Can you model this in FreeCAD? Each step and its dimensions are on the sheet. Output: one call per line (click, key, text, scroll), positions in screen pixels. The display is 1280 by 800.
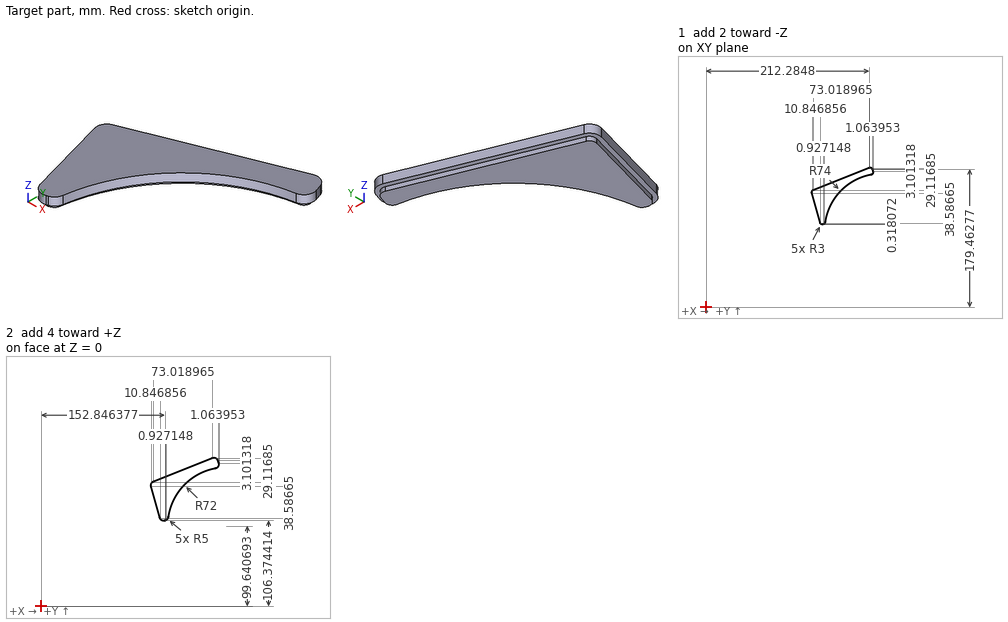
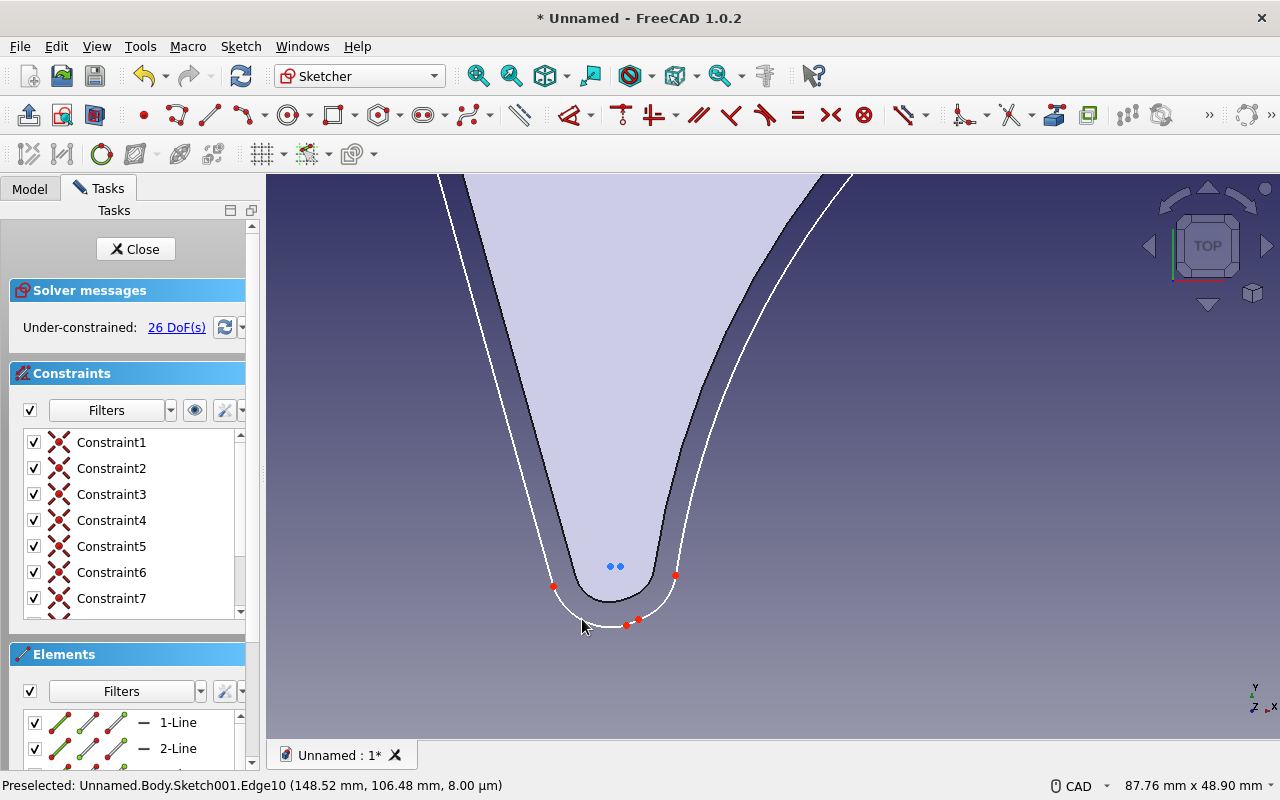
scroll(633, 622, up, 4)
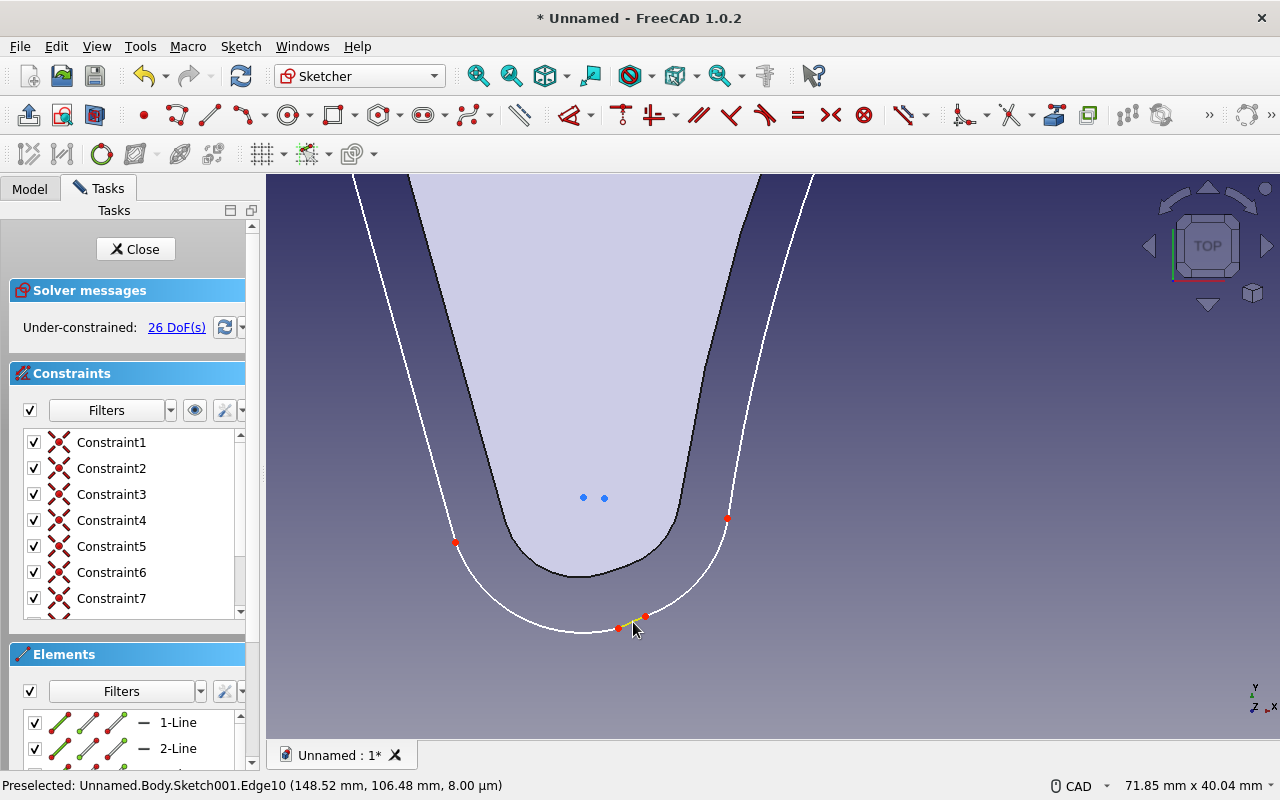
click(632, 622)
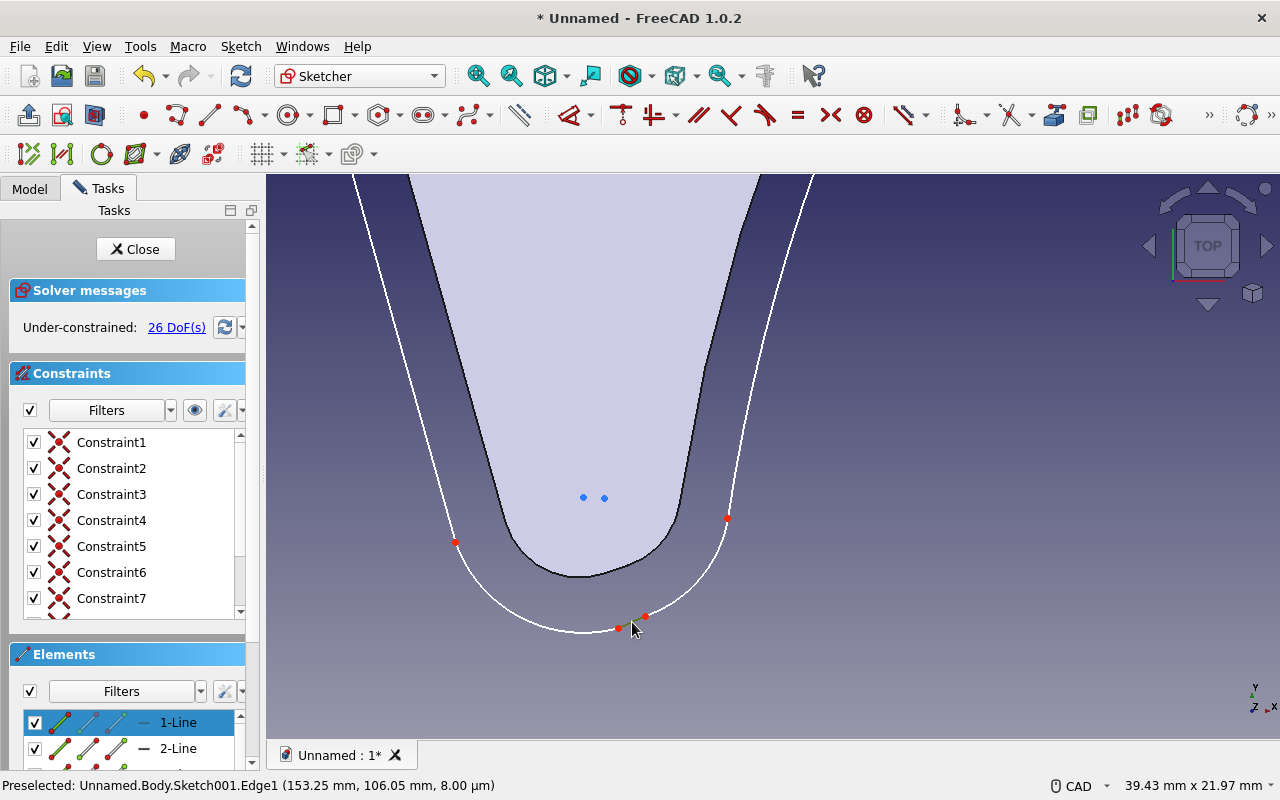
scroll(596, 620, down, 9)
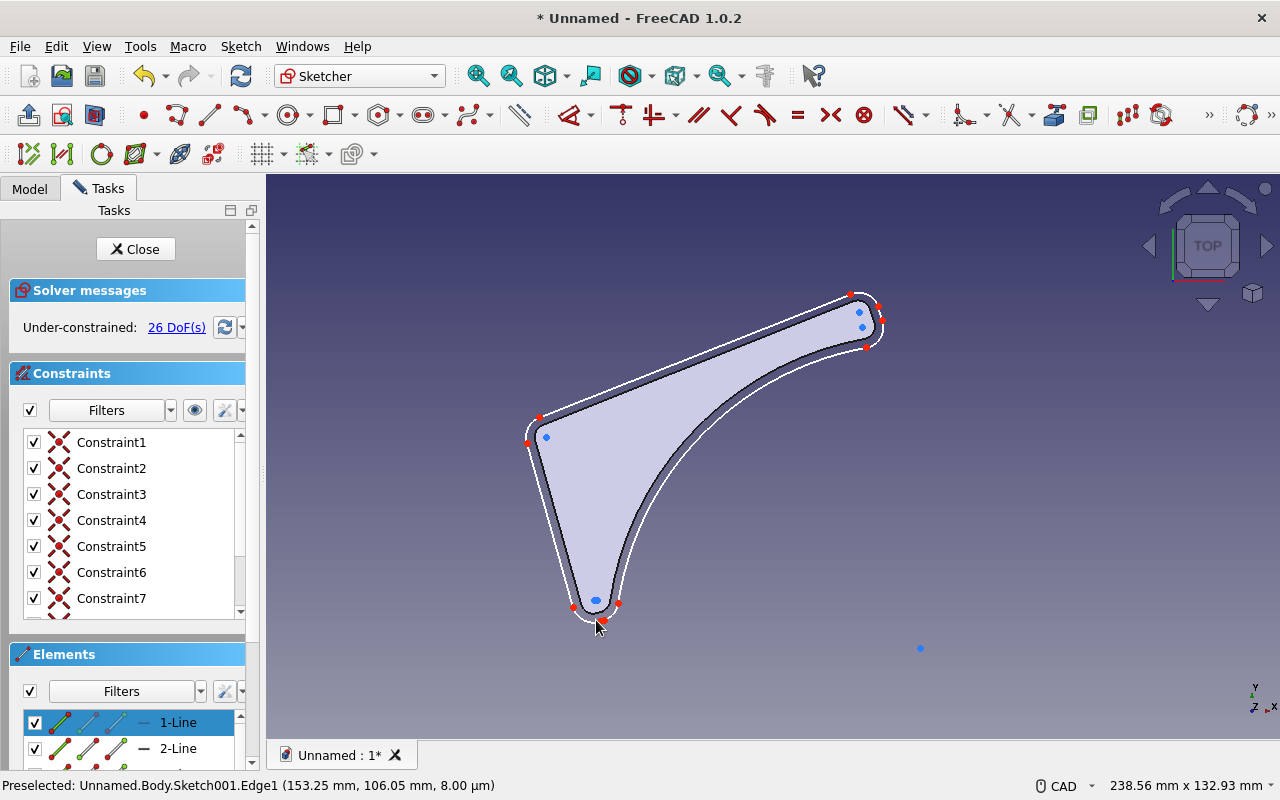
scroll(610, 617, up, 4)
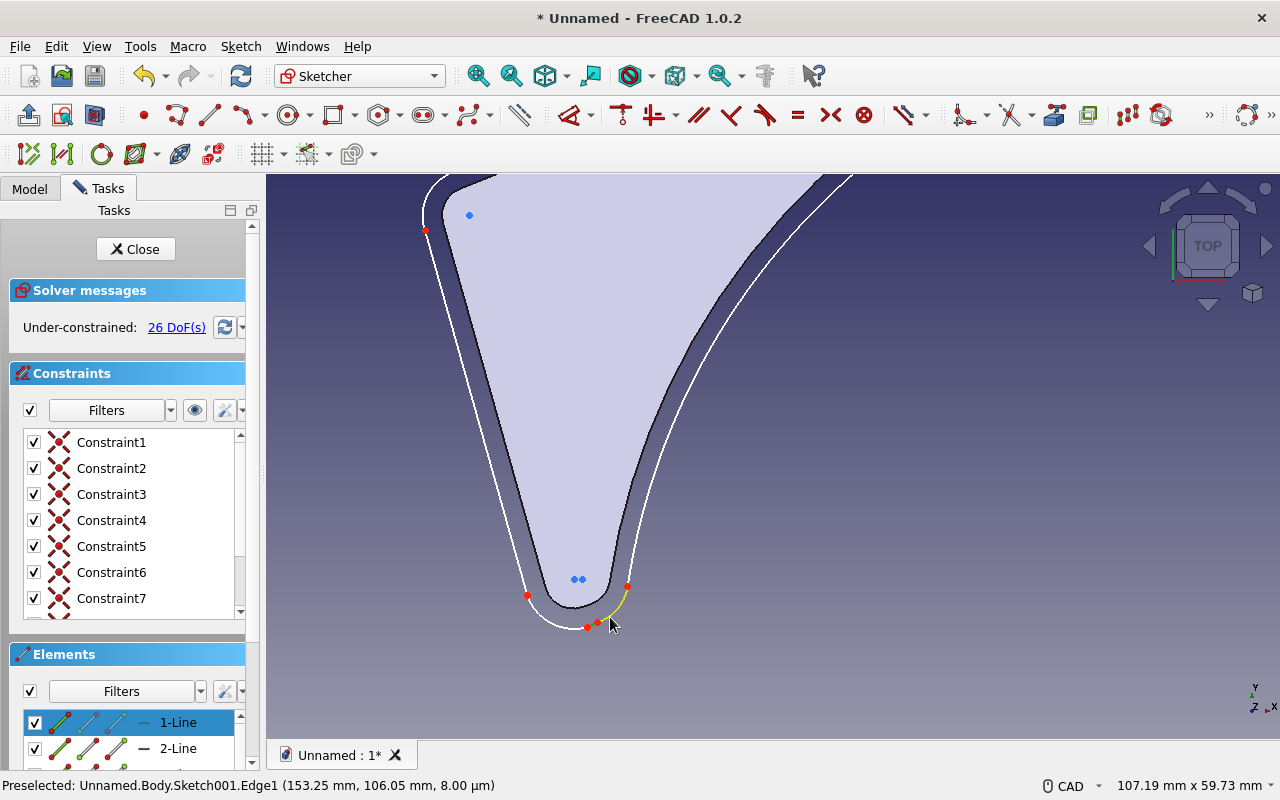
click(610, 616)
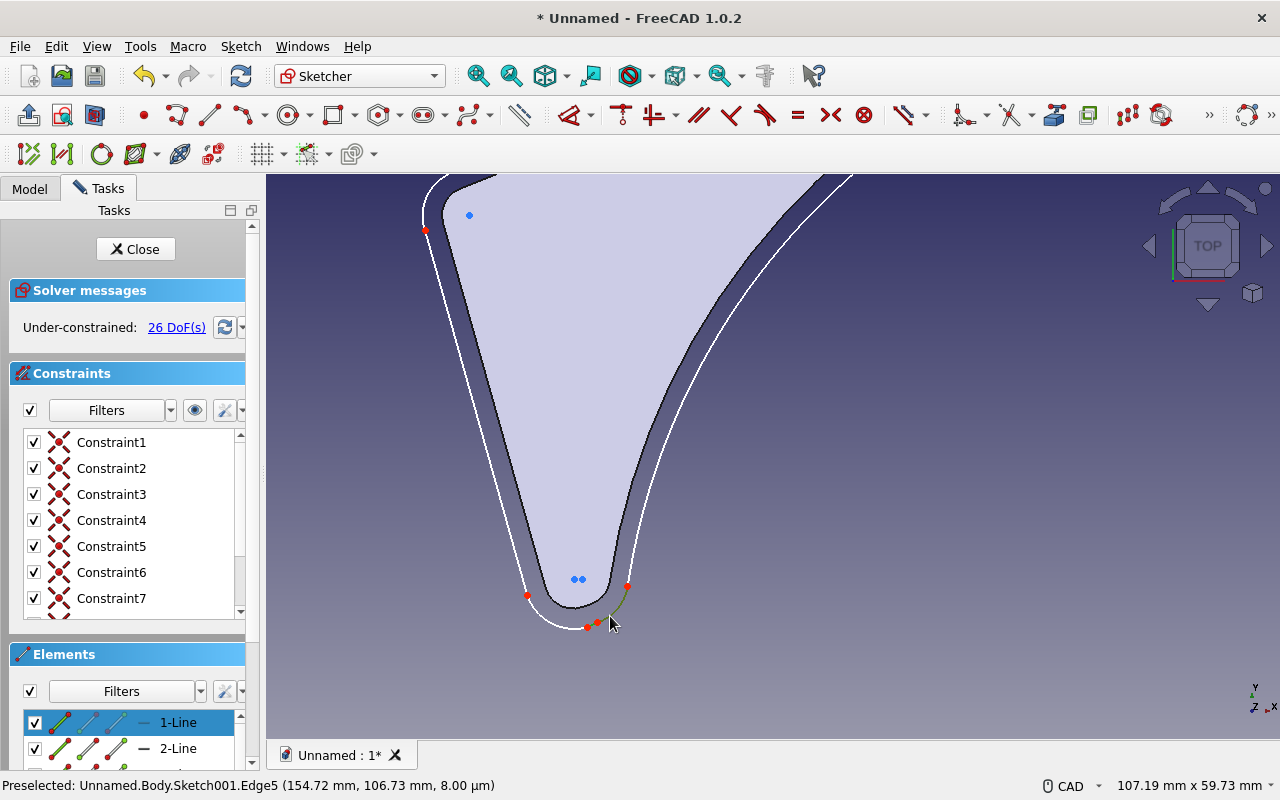
click(765, 116)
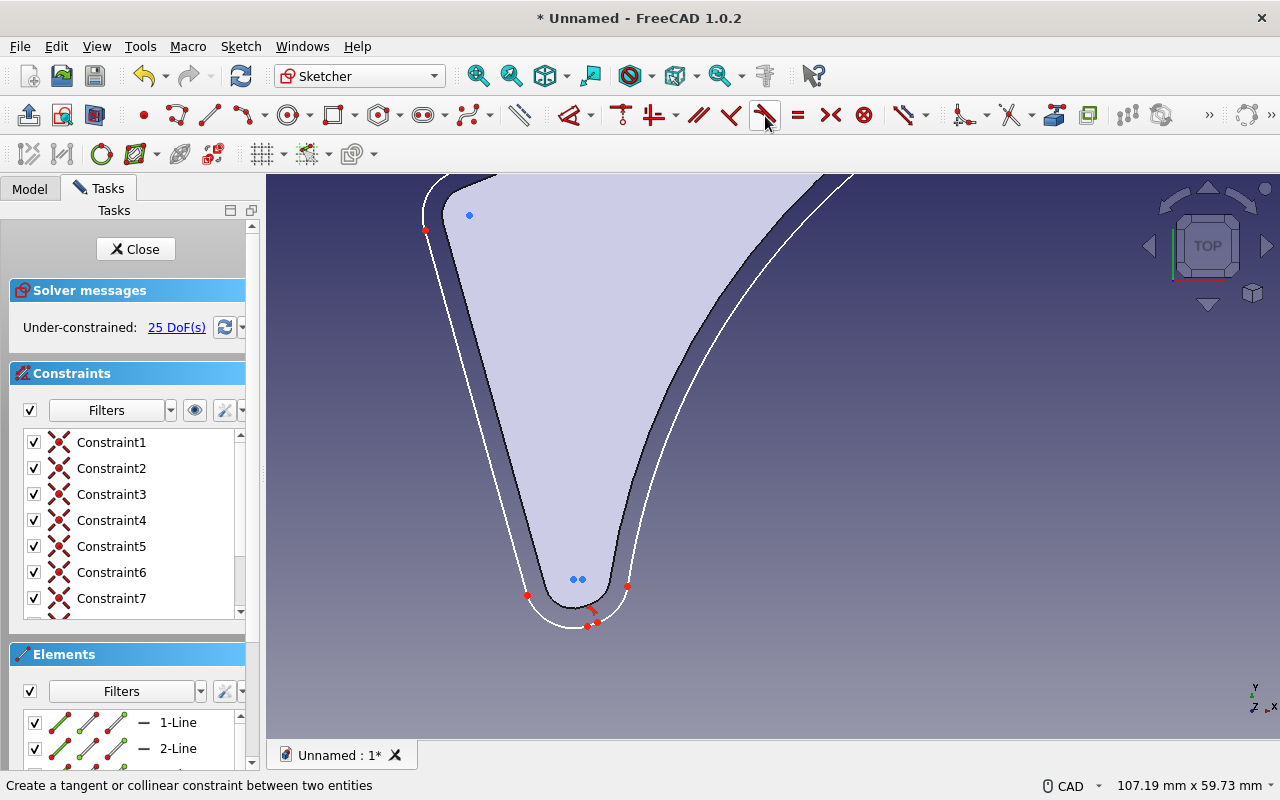
scroll(592, 625, up, 5)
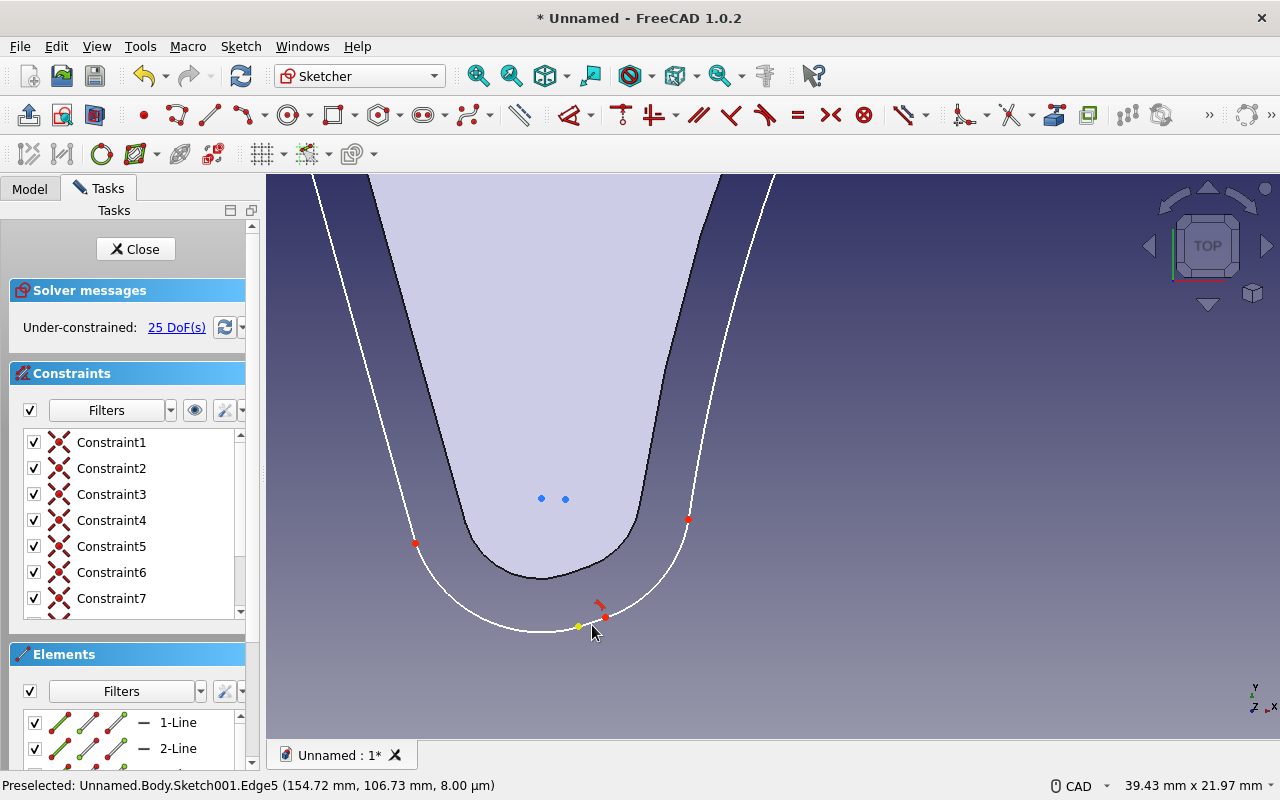
click(592, 622)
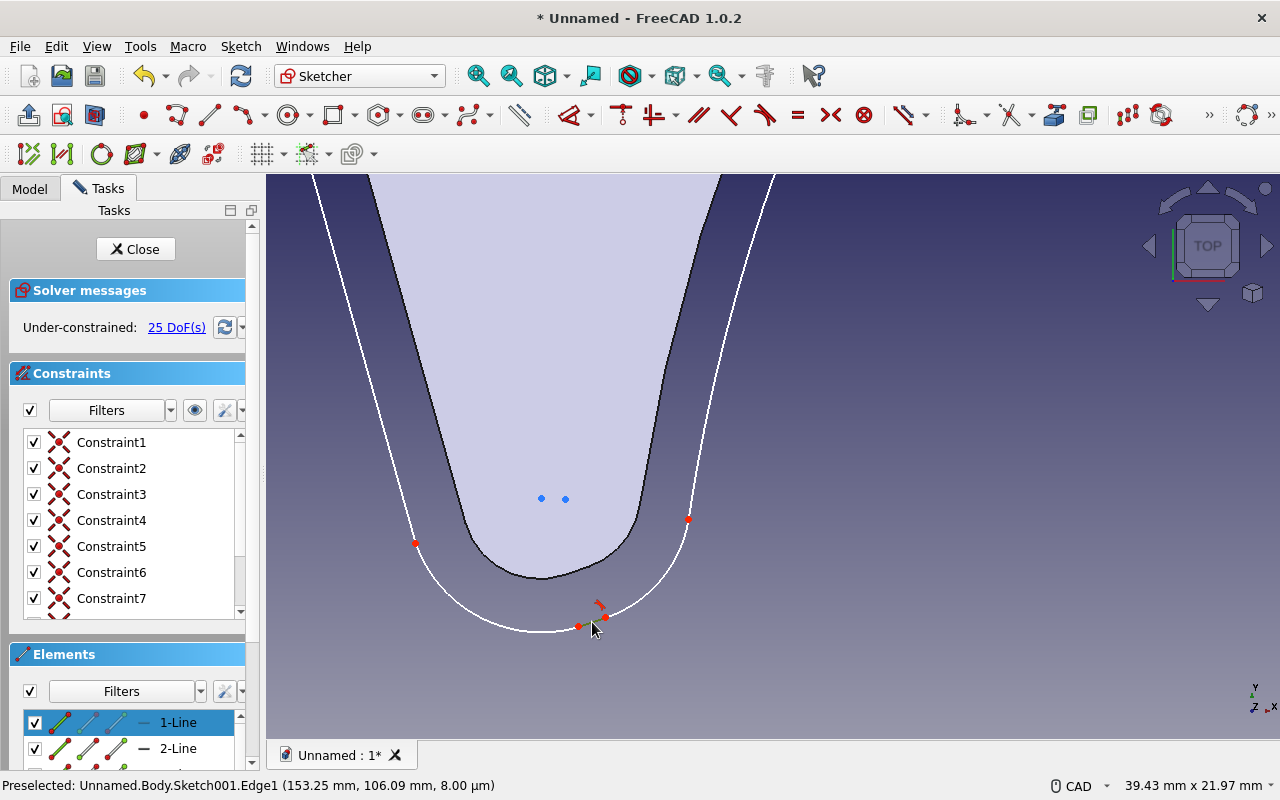
scroll(604, 620, down, 9)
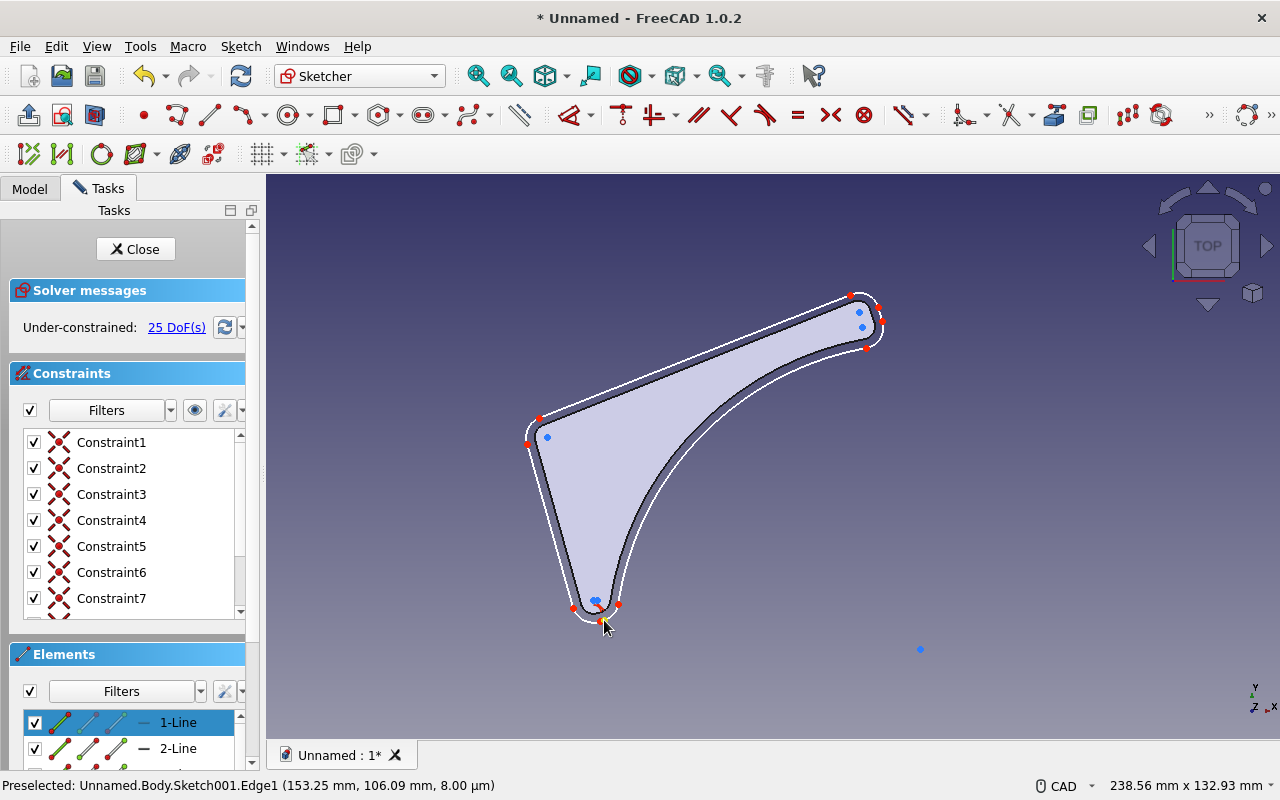
scroll(579, 616, up, 2)